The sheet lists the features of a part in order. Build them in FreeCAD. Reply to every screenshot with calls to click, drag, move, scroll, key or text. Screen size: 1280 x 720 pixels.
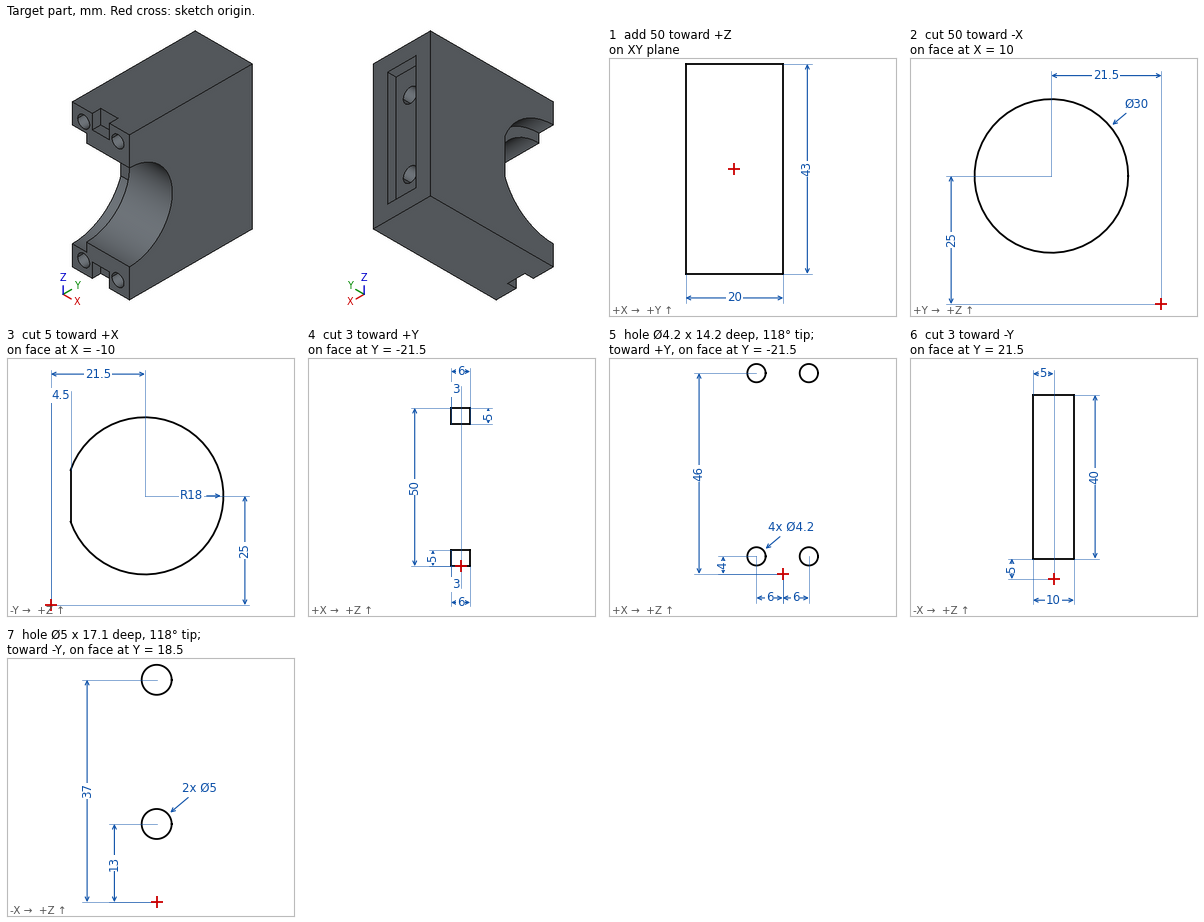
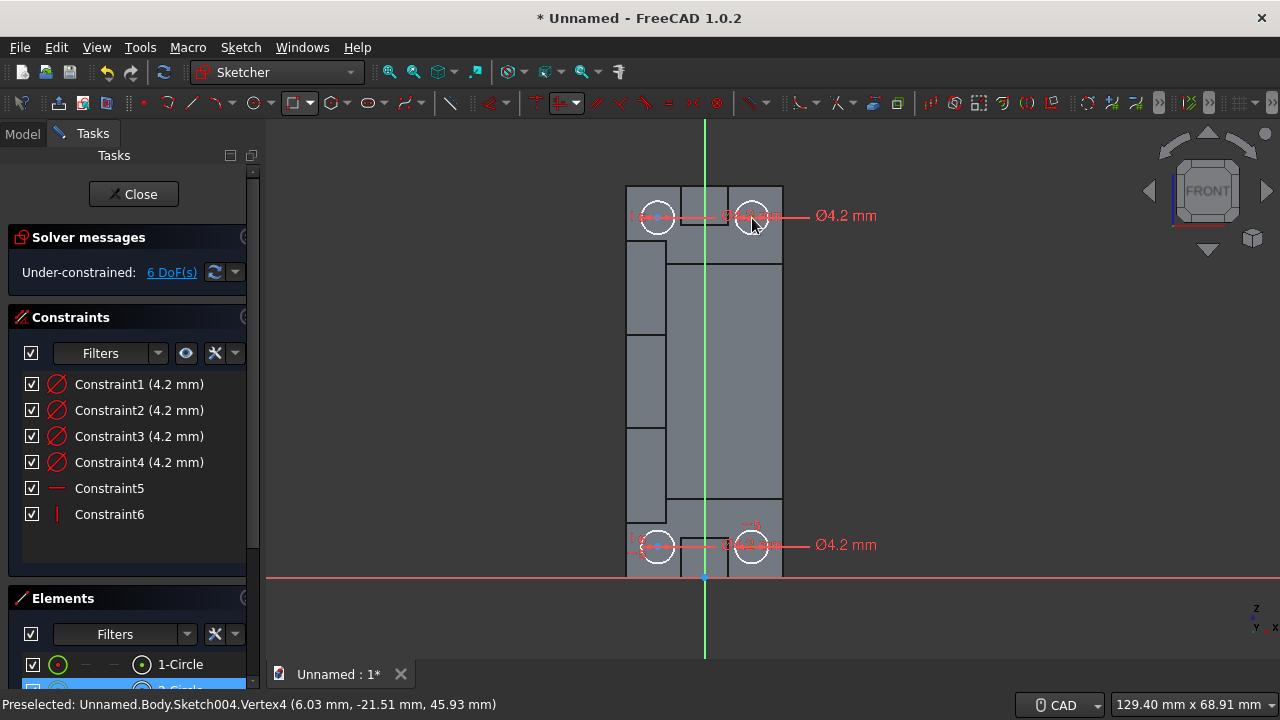
key(v)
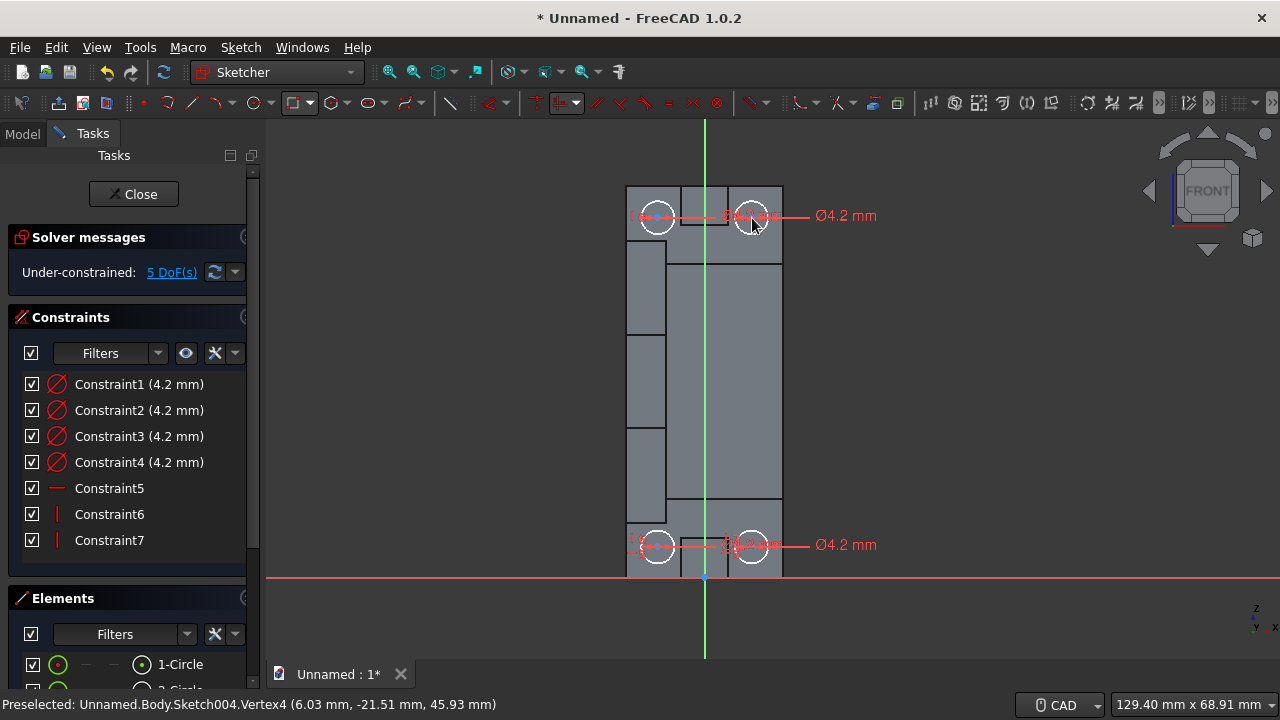
click(658, 218)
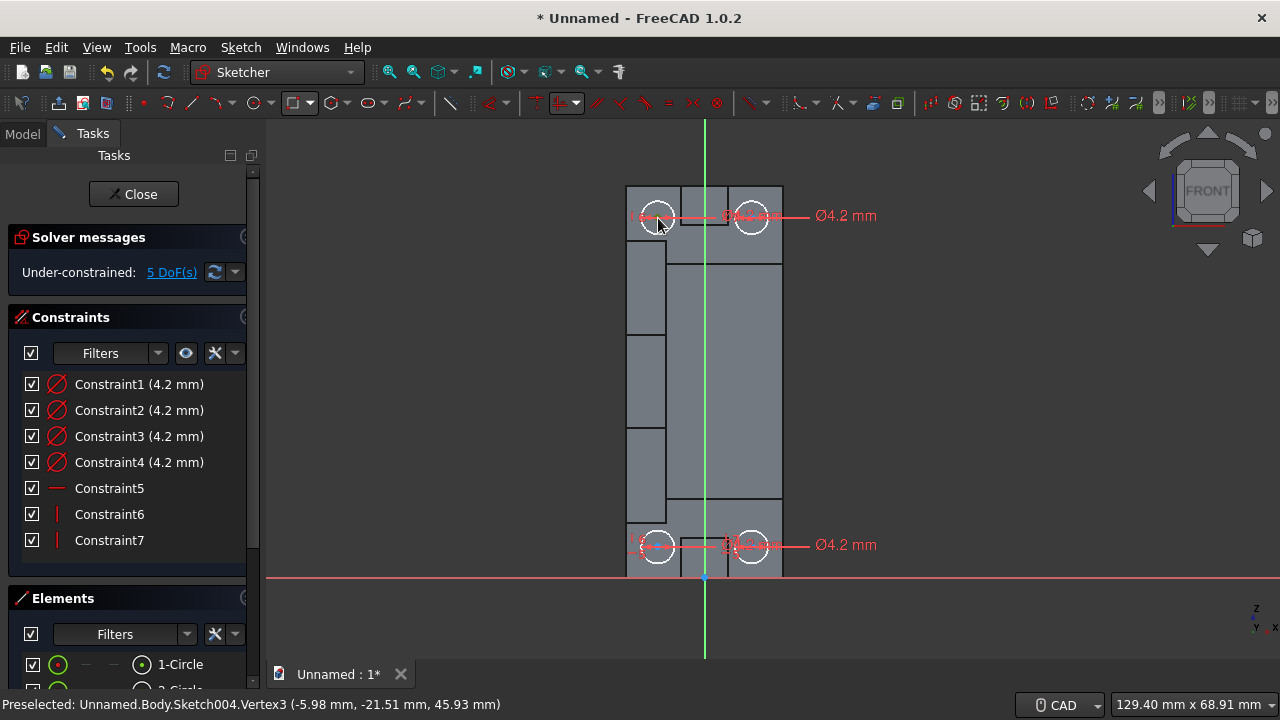
click(752, 218)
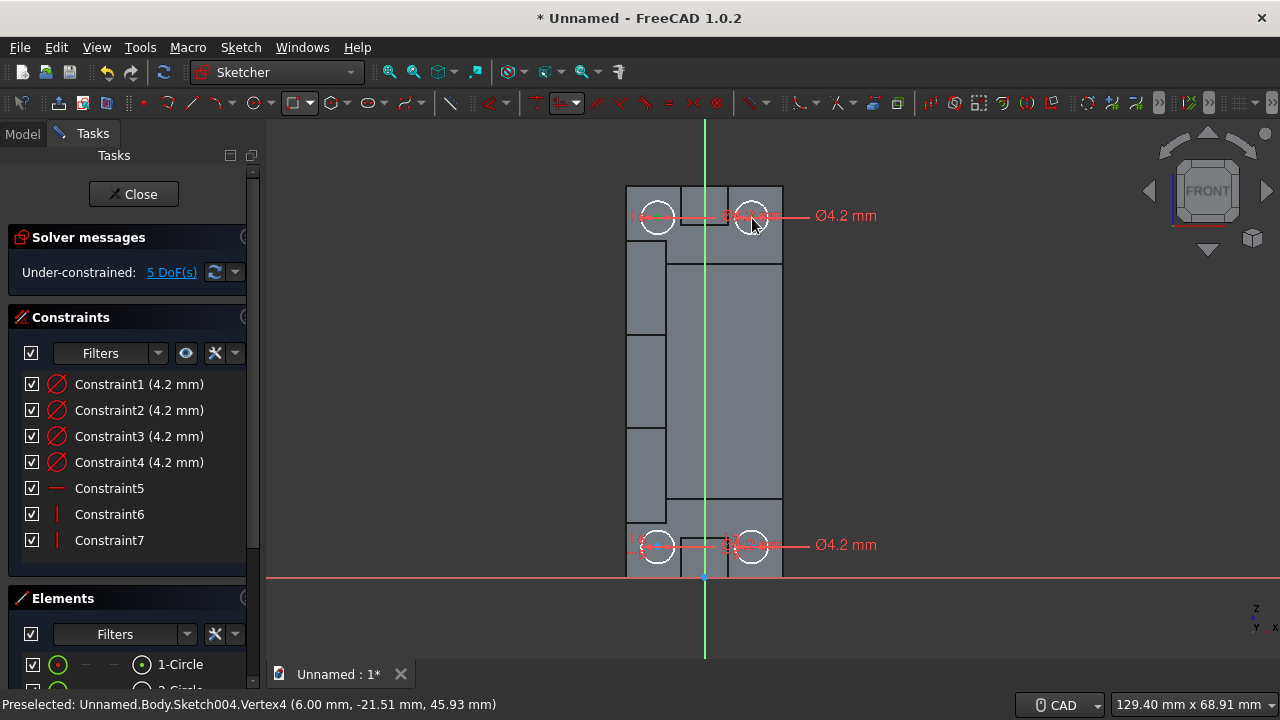
key(h)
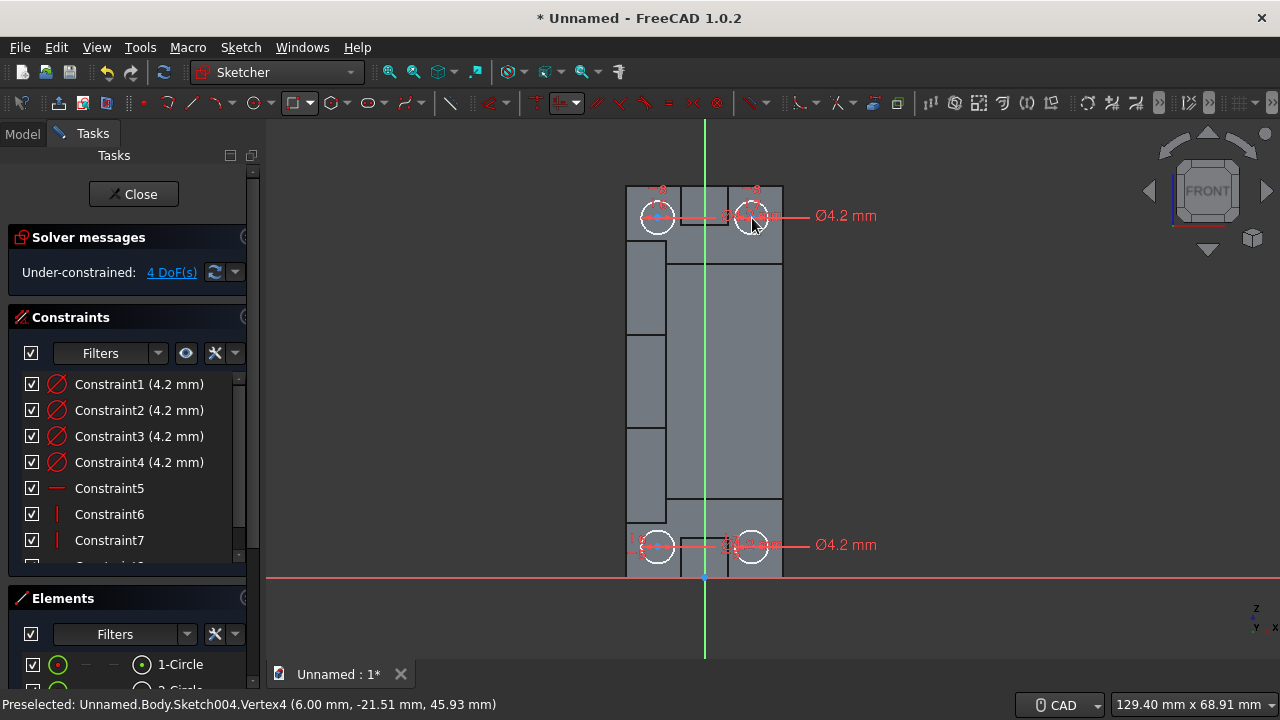
click(490, 104)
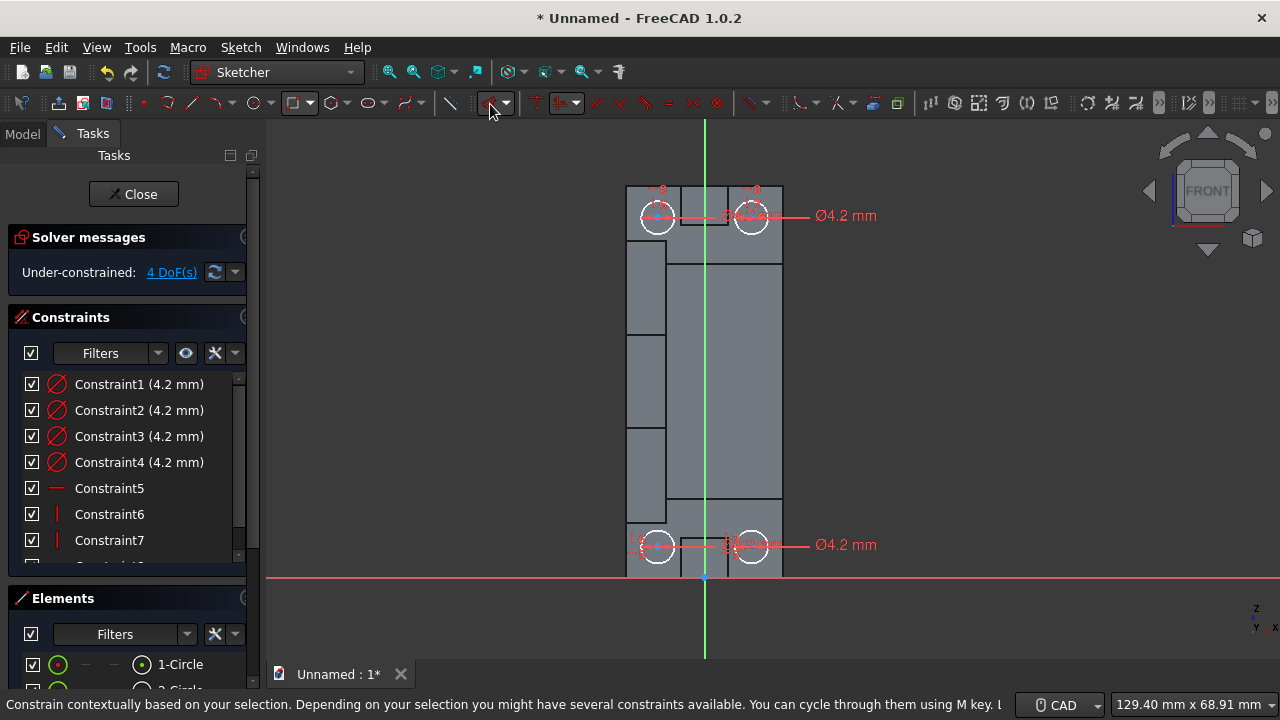
click(658, 547)
click(681, 612)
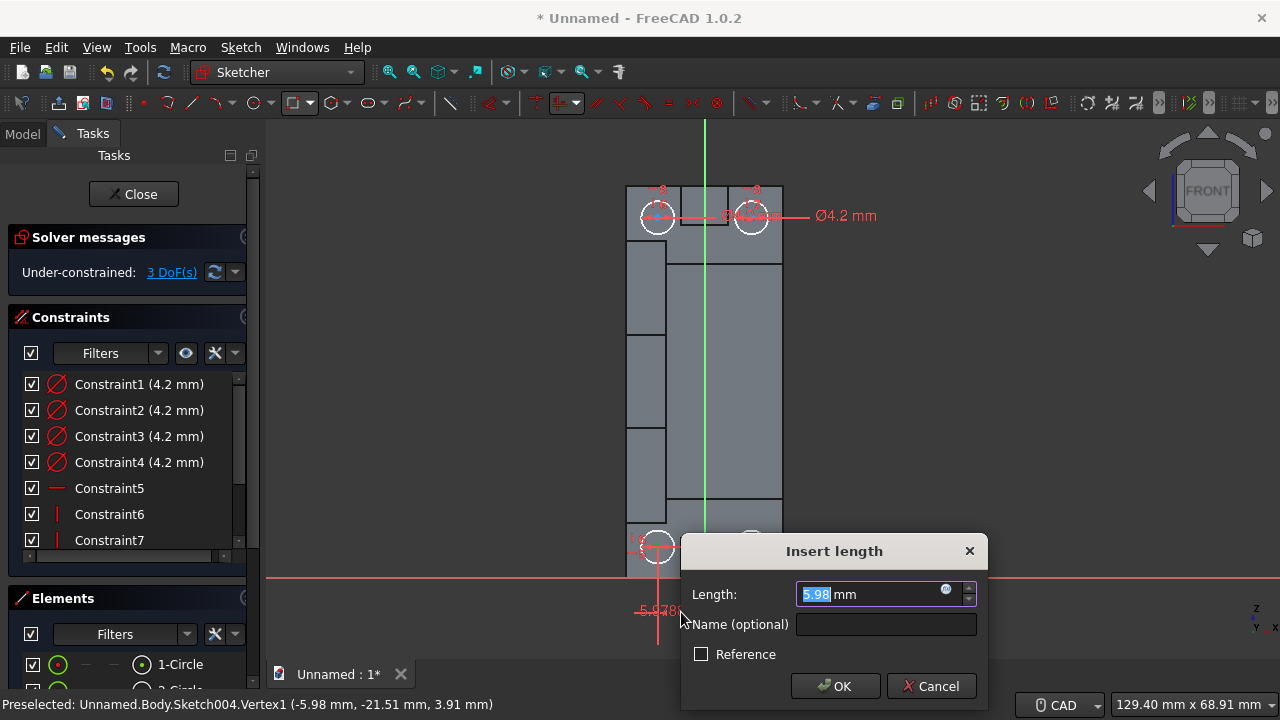
text(6)
key(Return)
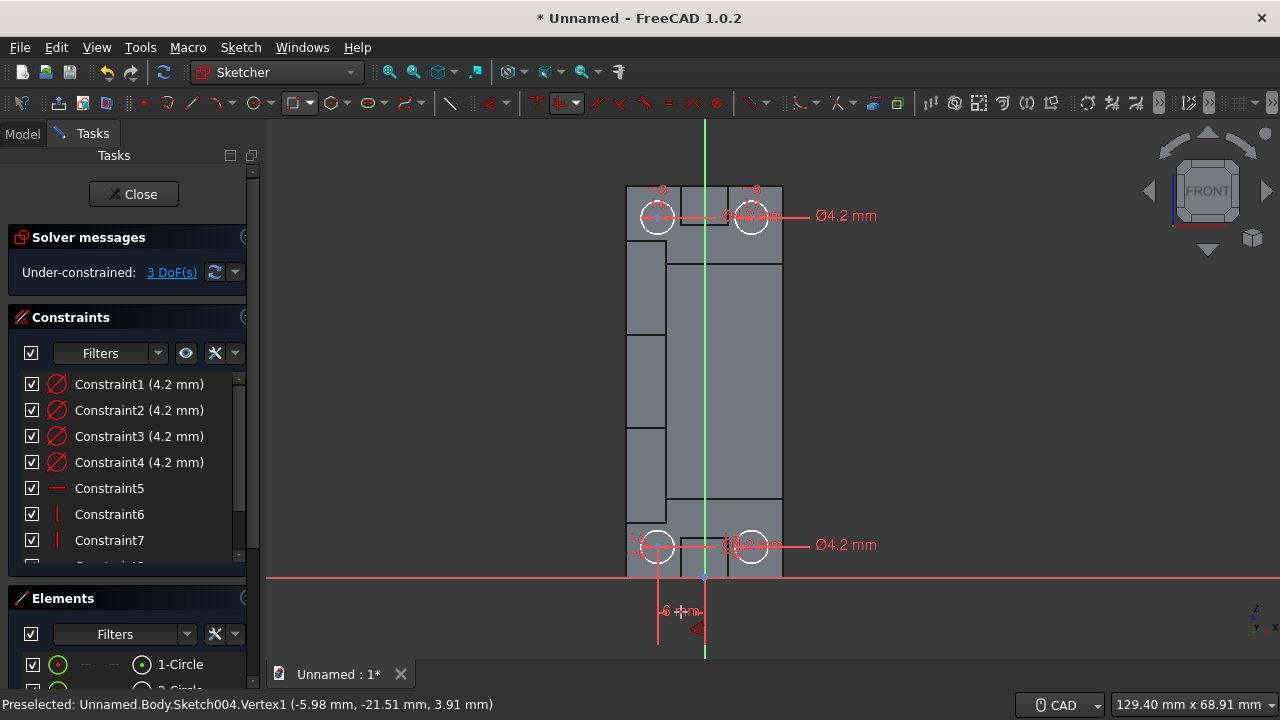
scroll(658, 547, up, 2)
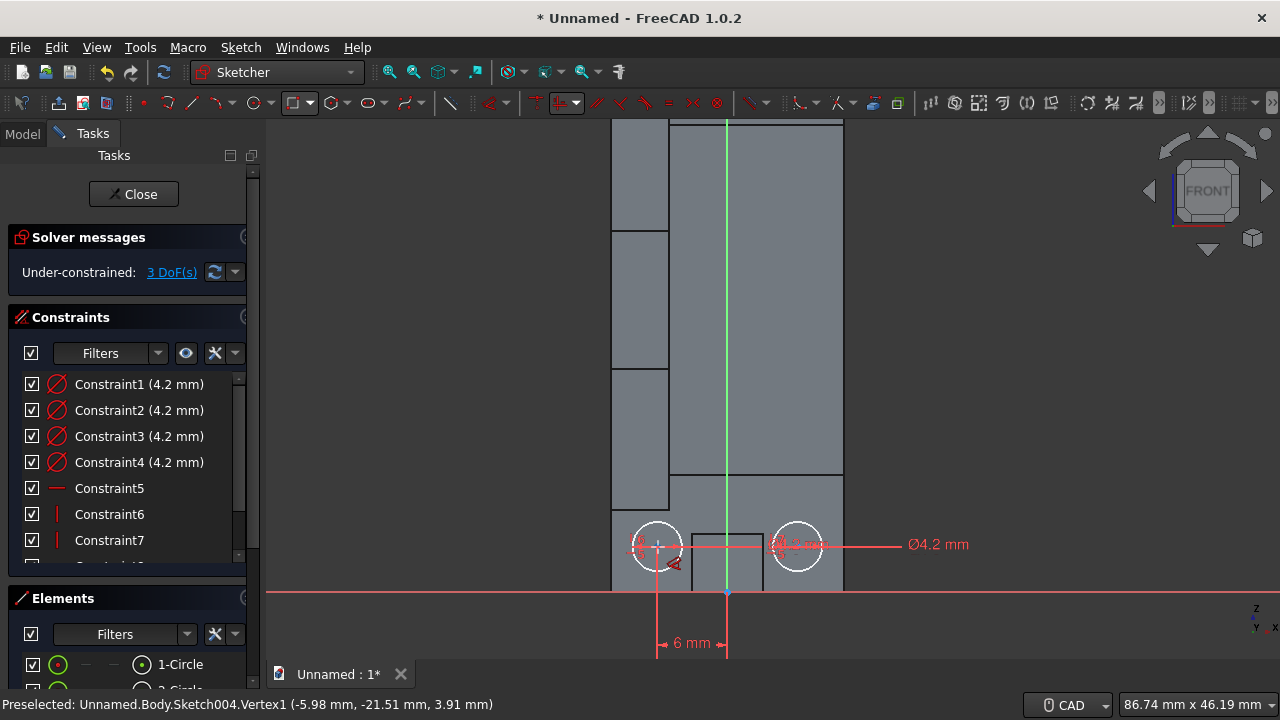
click(657, 547)
click(623, 569)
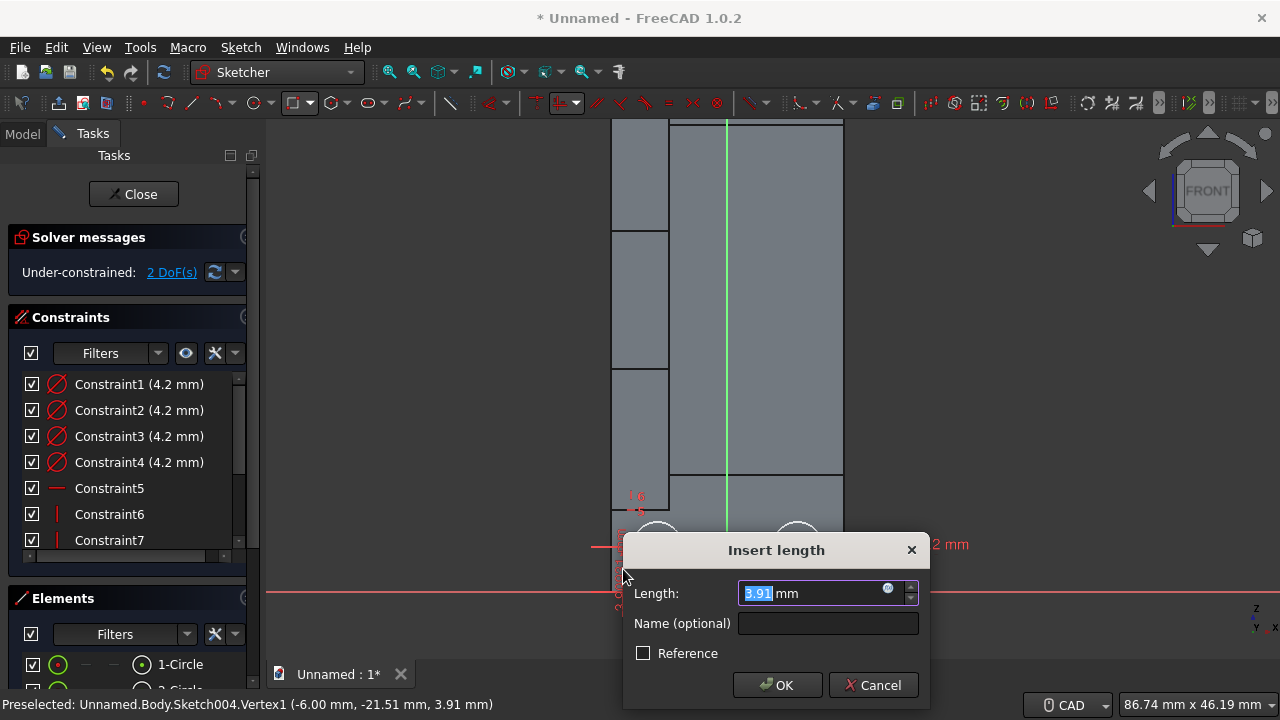
text(4)
key(Return)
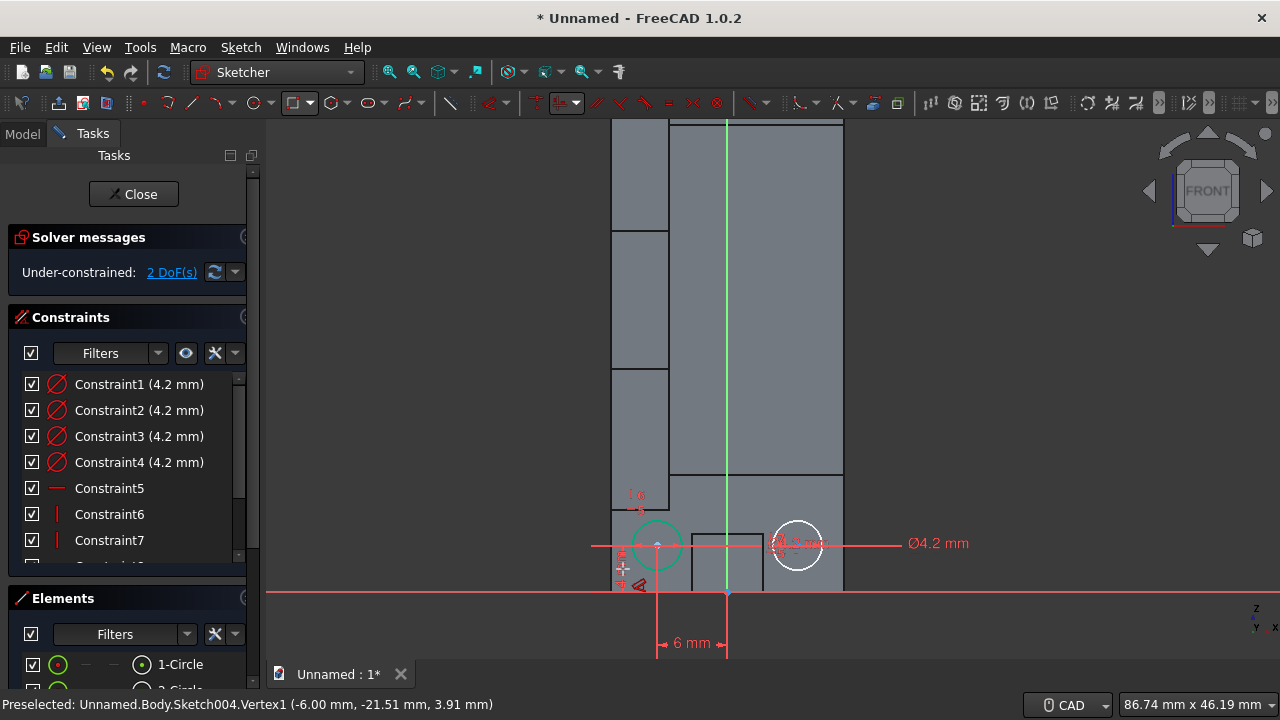
click(798, 546)
click(779, 626)